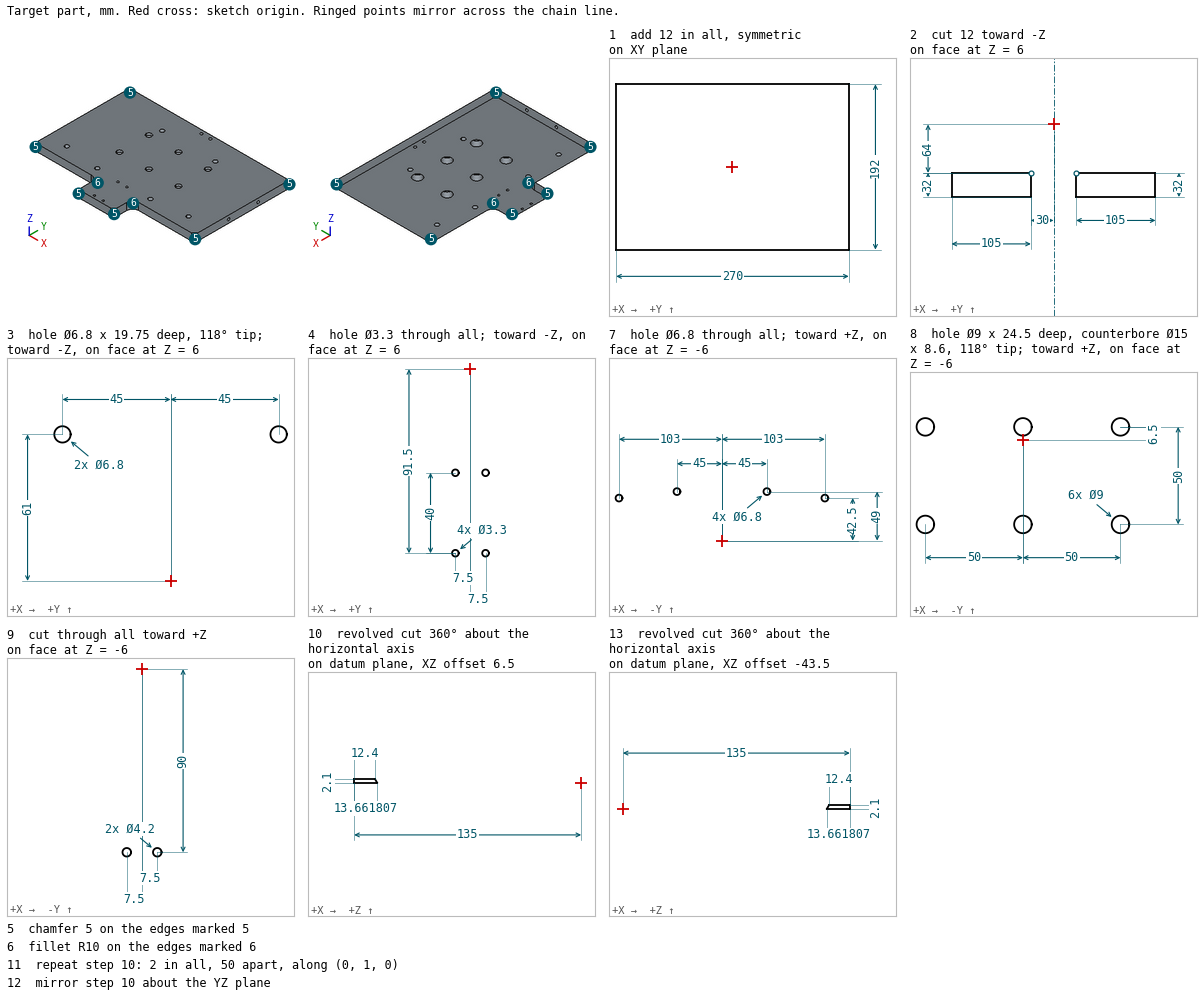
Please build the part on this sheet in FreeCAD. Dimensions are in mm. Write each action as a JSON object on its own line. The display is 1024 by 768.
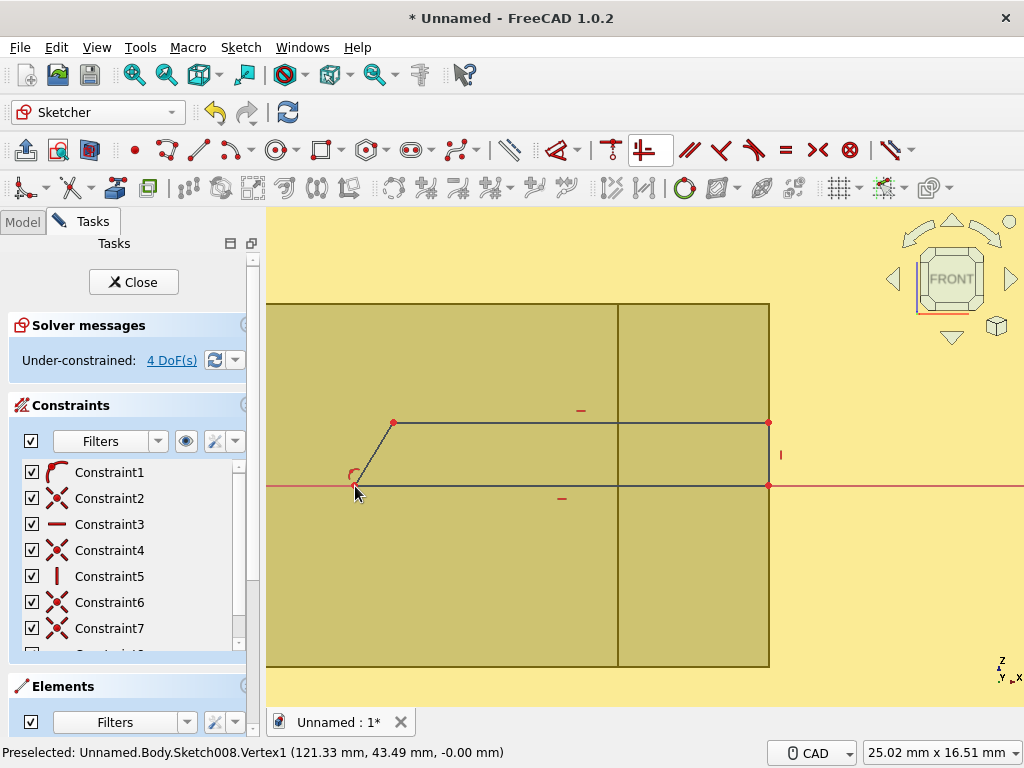
{"action": "key", "text": "d"}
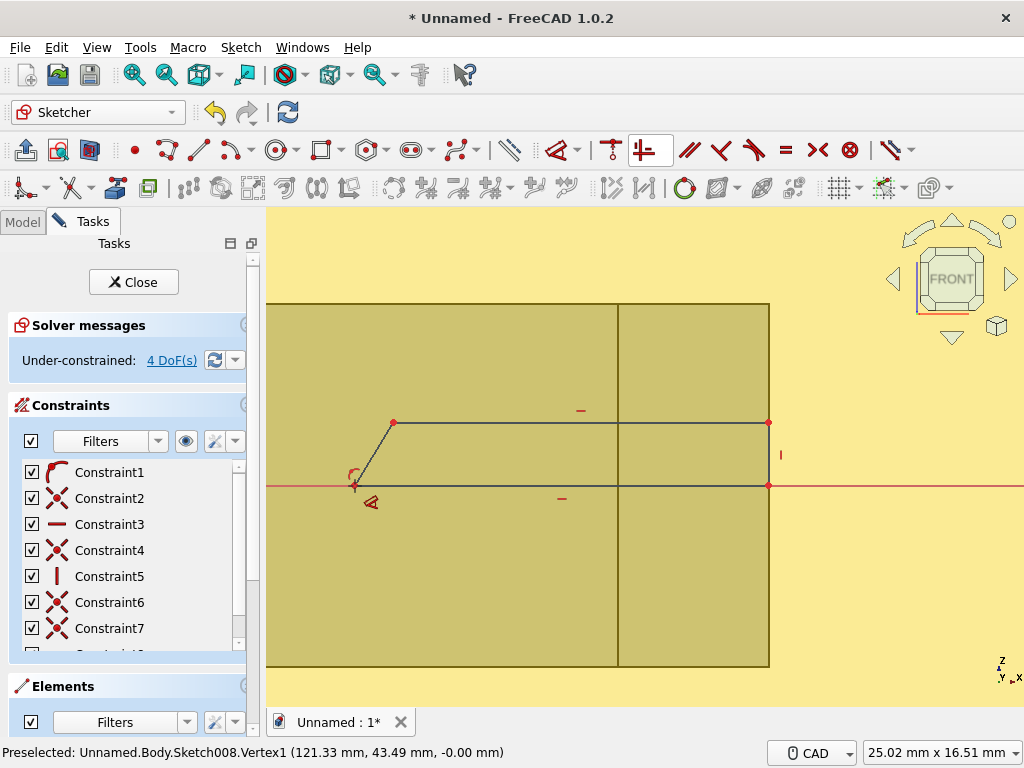
{"action": "left_click", "coordinate": [769, 442]}
{"action": "left_click", "coordinate": [803, 454]}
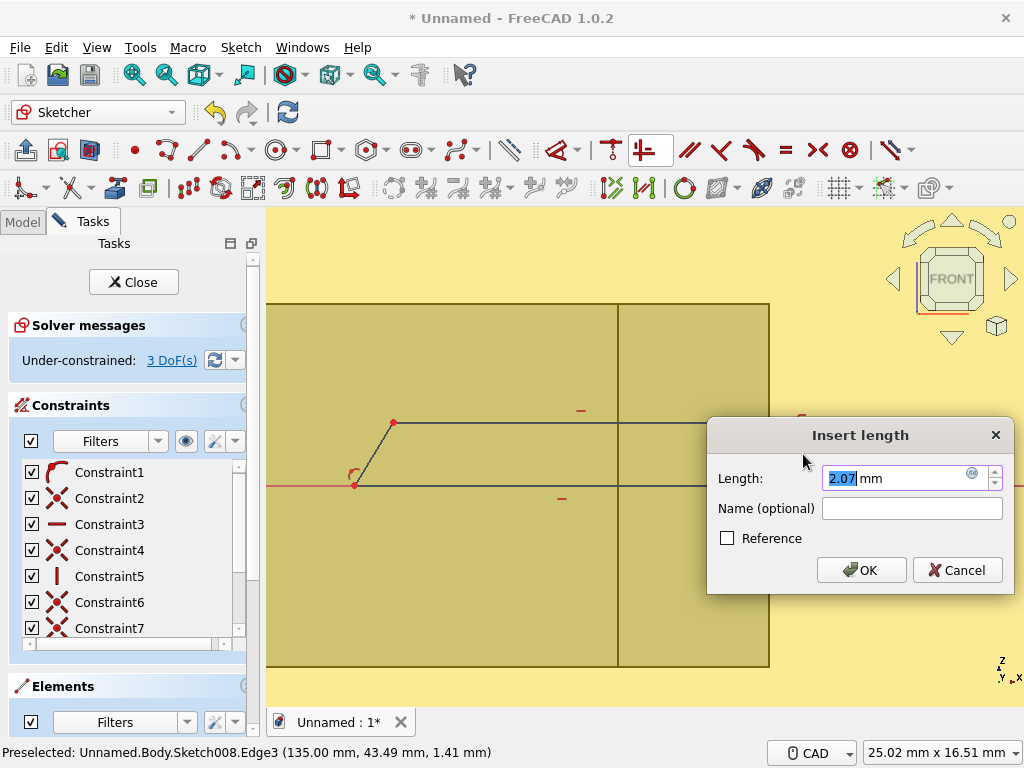
{"action": "type", "text": "2.1"}
{"action": "key", "text": "Return"}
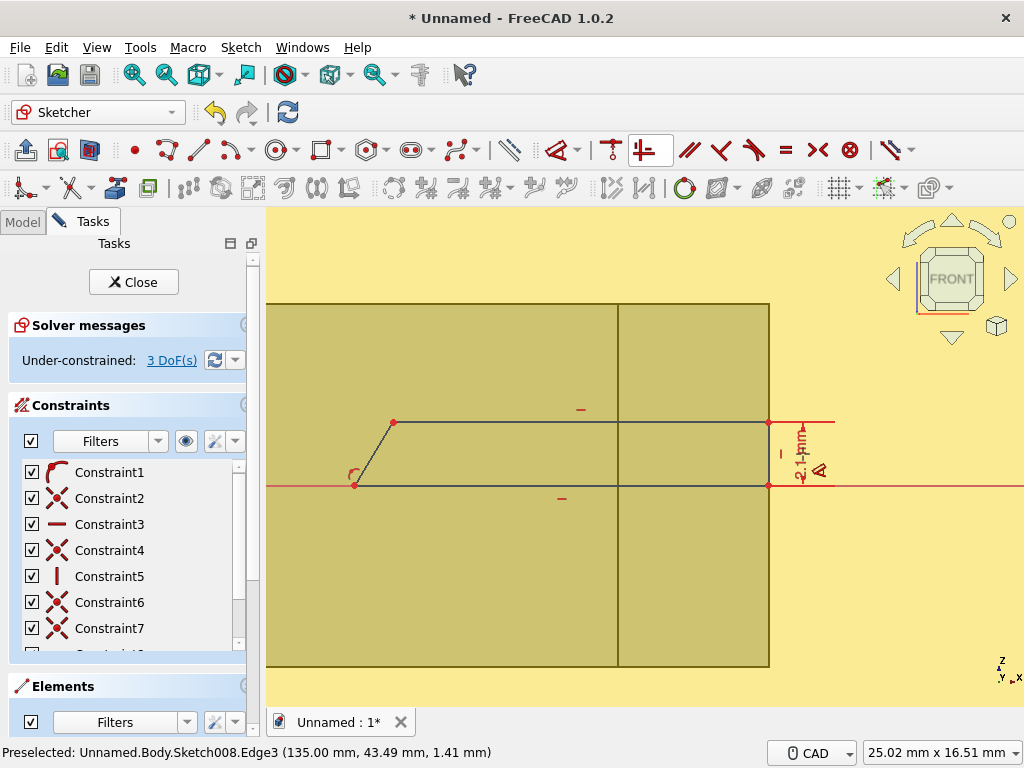
{"action": "left_click", "coordinate": [506, 422]}
{"action": "left_click", "coordinate": [581, 388]}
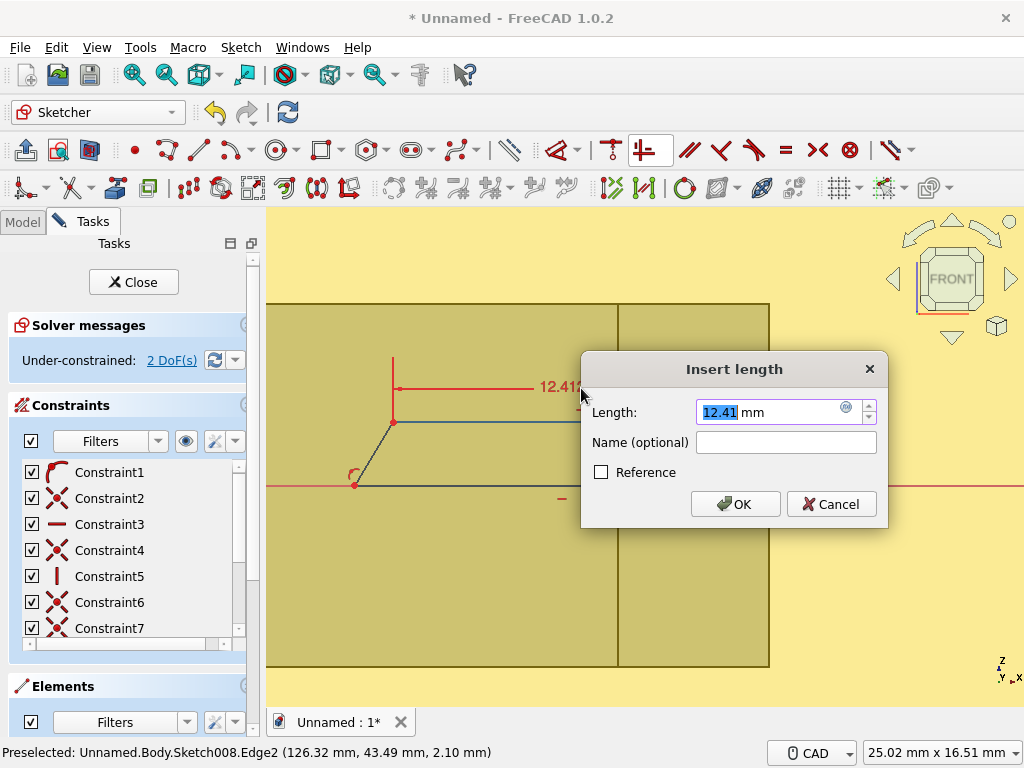
{"action": "type", "text": "12.4"}
{"action": "key", "text": "Return"}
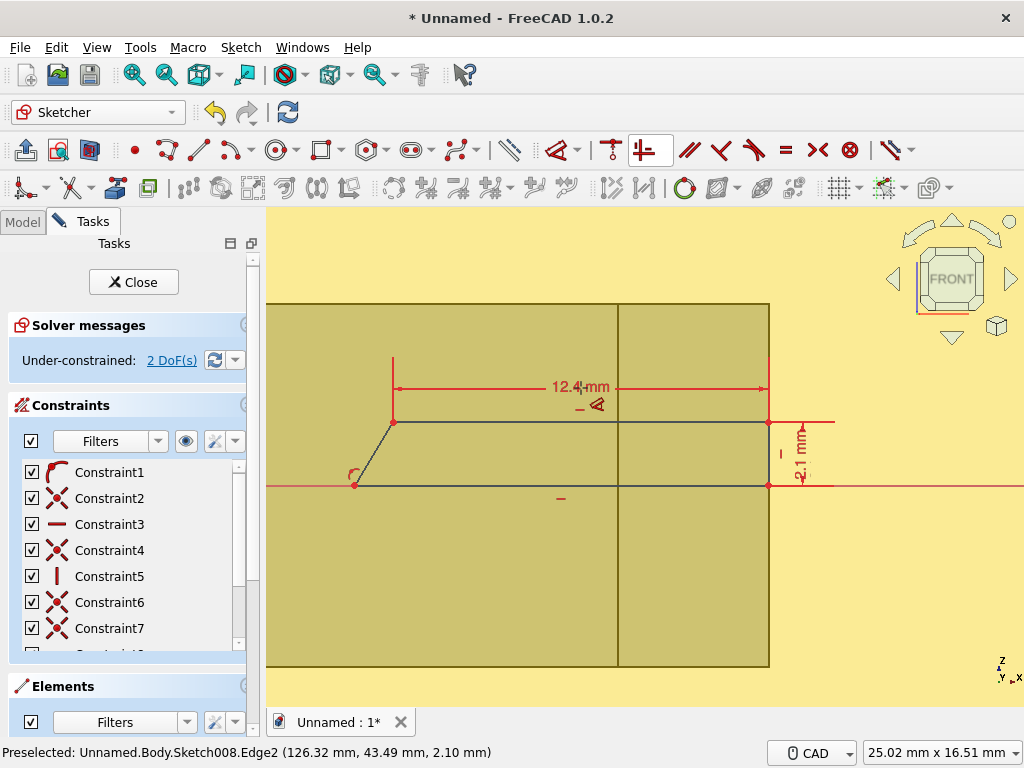
{"action": "left_click", "coordinate": [769, 422]}
{"action": "left_click", "coordinate": [422, 388]}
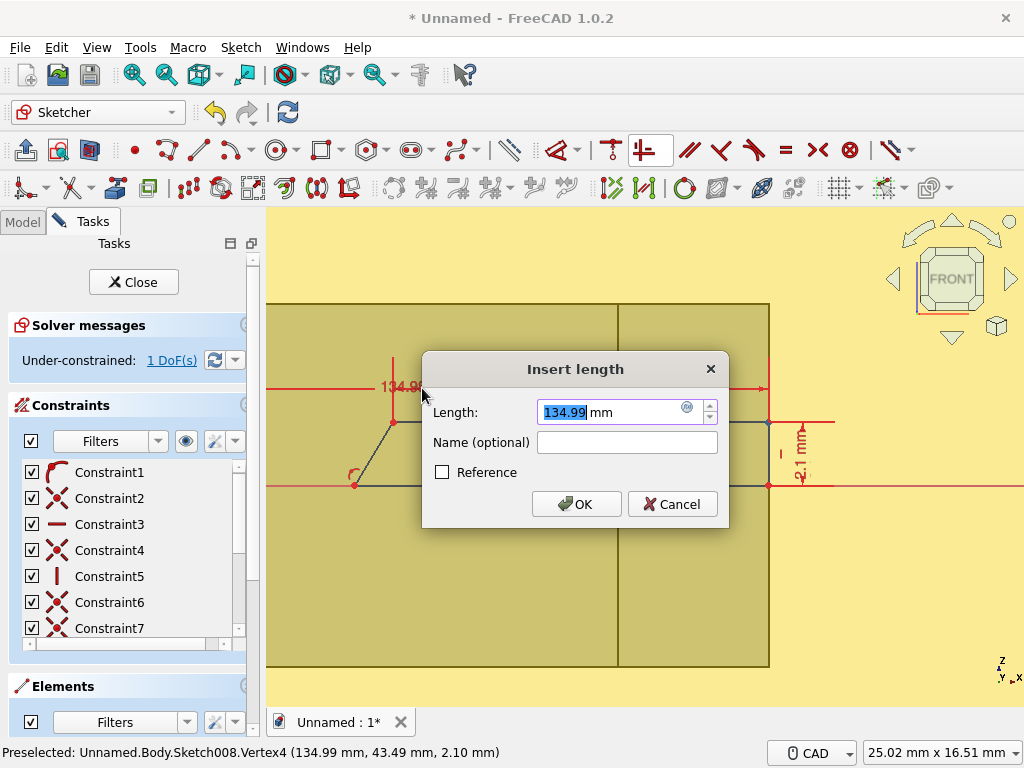
{"action": "type", "text": "135"}
{"action": "key", "text": "Return"}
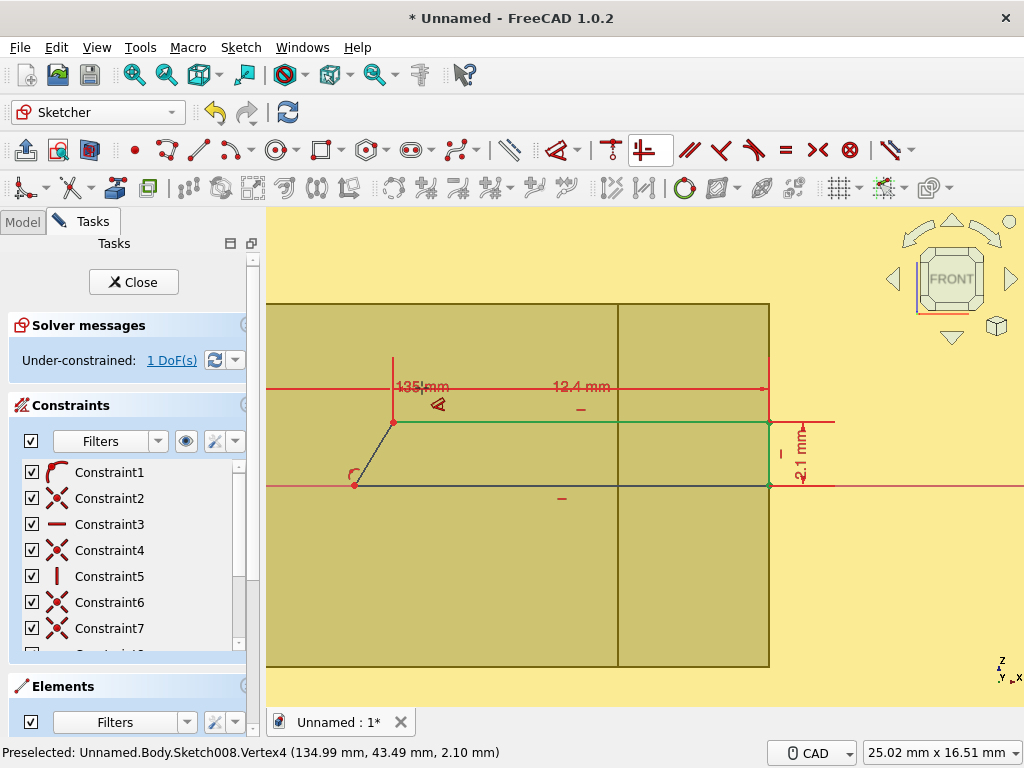
{"action": "left_click", "coordinate": [645, 486]}
{"action": "left_click", "coordinate": [562, 520]}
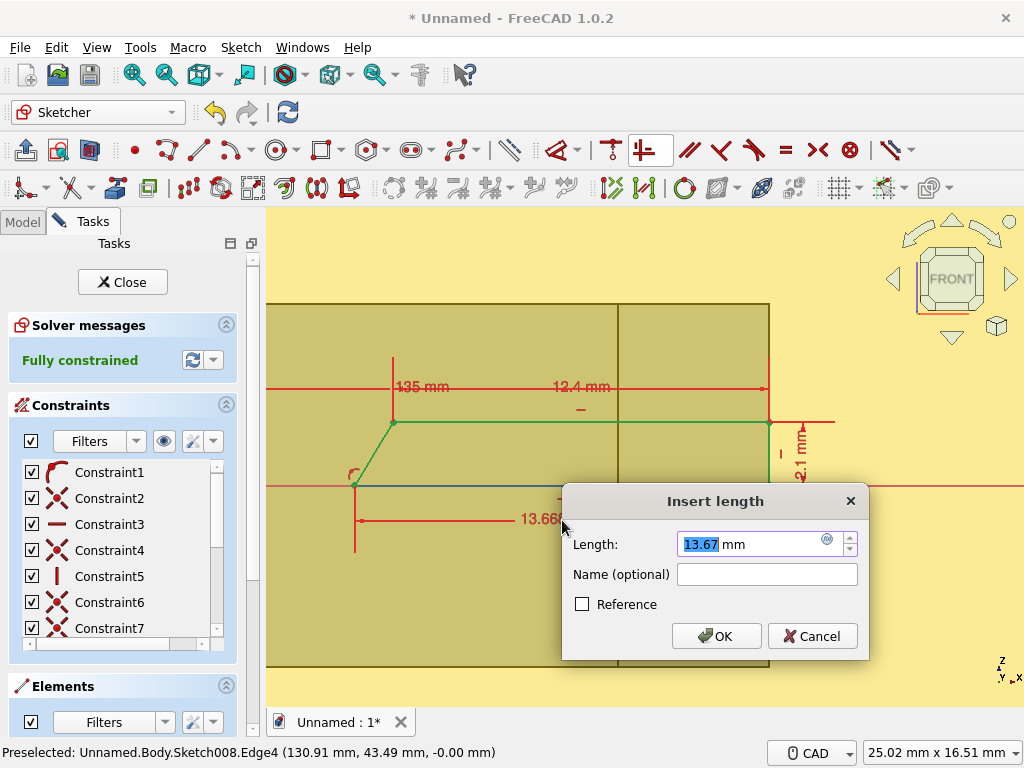
{"action": "type", "text": "13.661807"}
{"action": "key", "text": "Return"}
{"action": "key", "text": "Escape"}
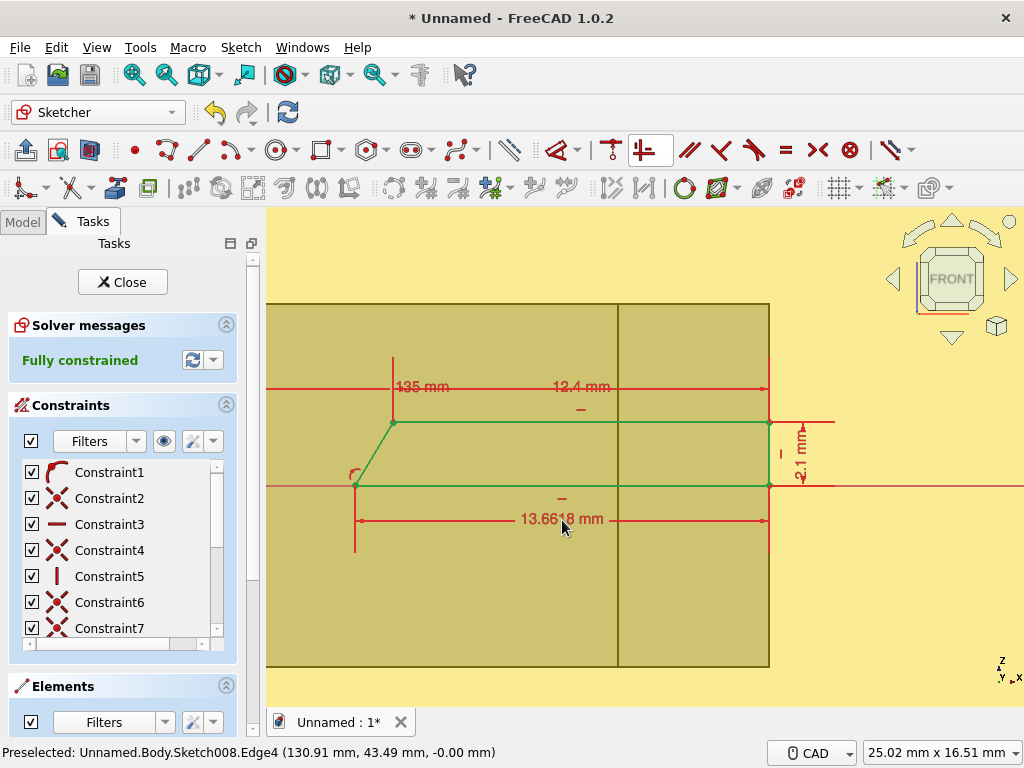
{"action": "left_click", "coordinate": [123, 282]}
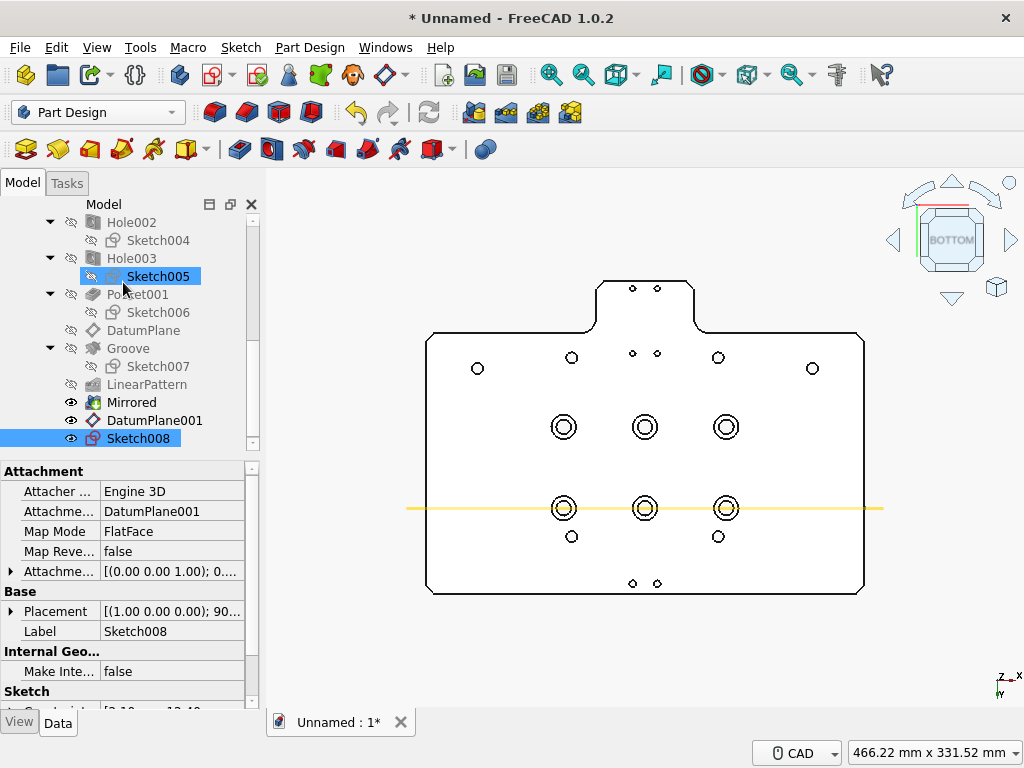
{"action": "left_click", "coordinate": [304, 150]}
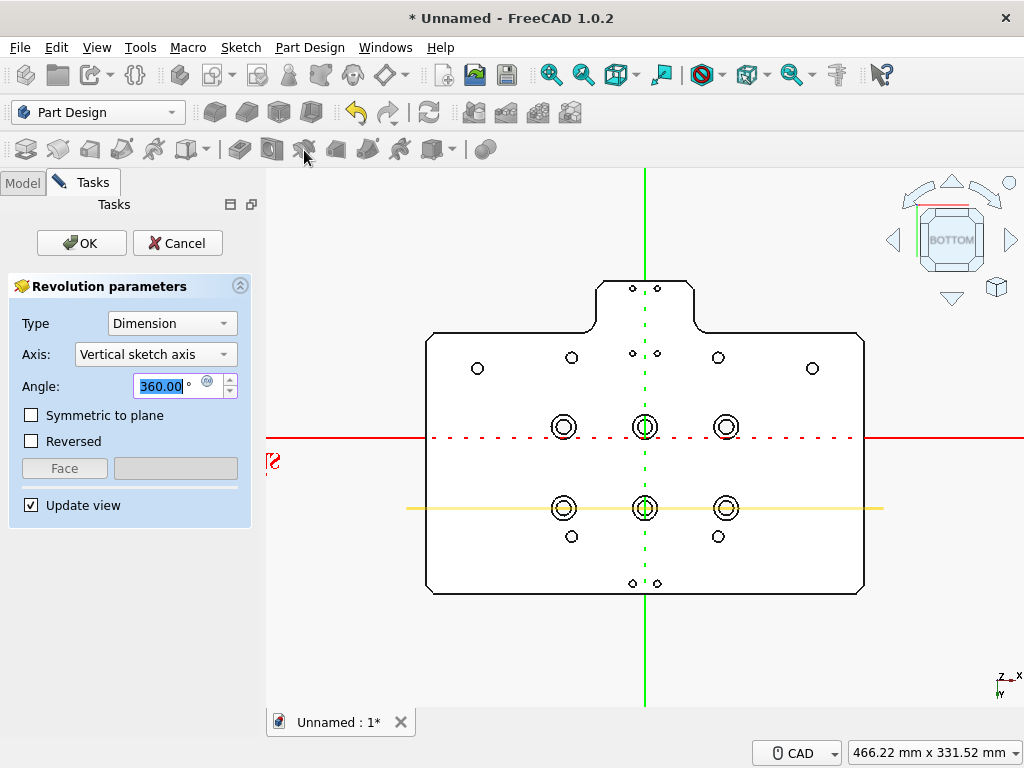
{"action": "left_click", "coordinate": [156, 354]}